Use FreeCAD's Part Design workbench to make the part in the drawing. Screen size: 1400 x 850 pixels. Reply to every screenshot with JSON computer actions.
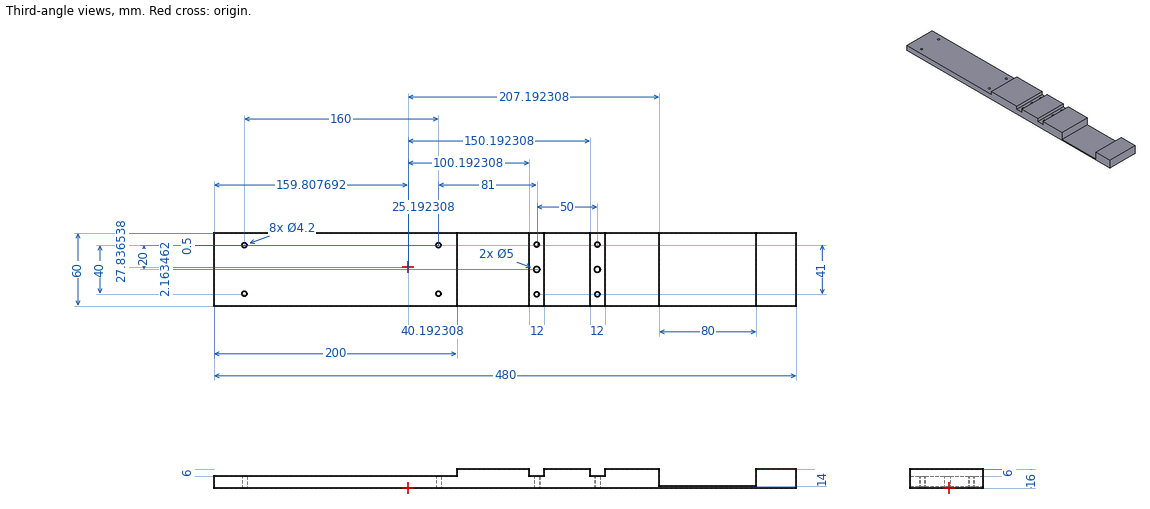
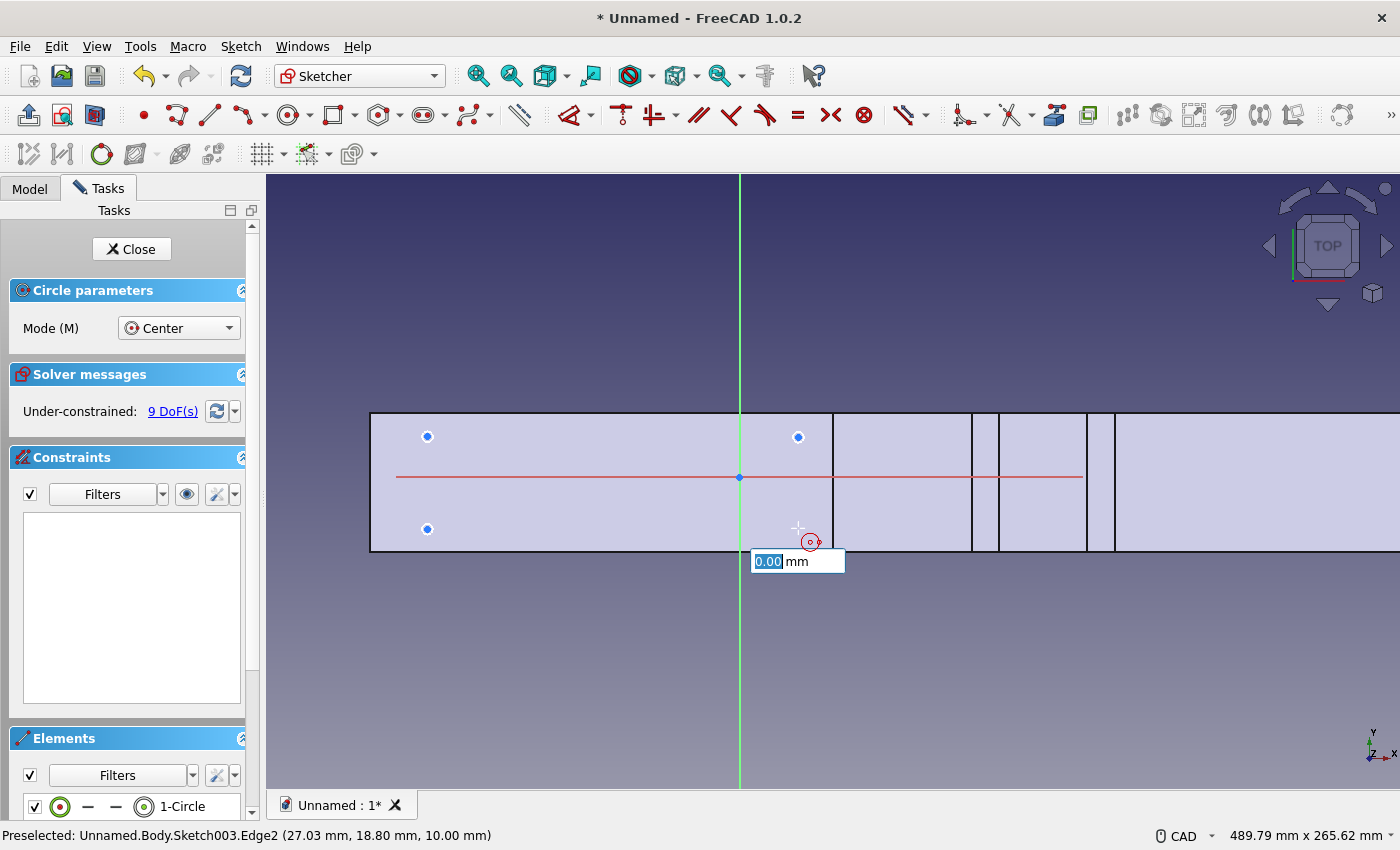
{"action": "scroll", "coordinate": [801, 525], "scroll_direction": "up", "scroll_amount": 6}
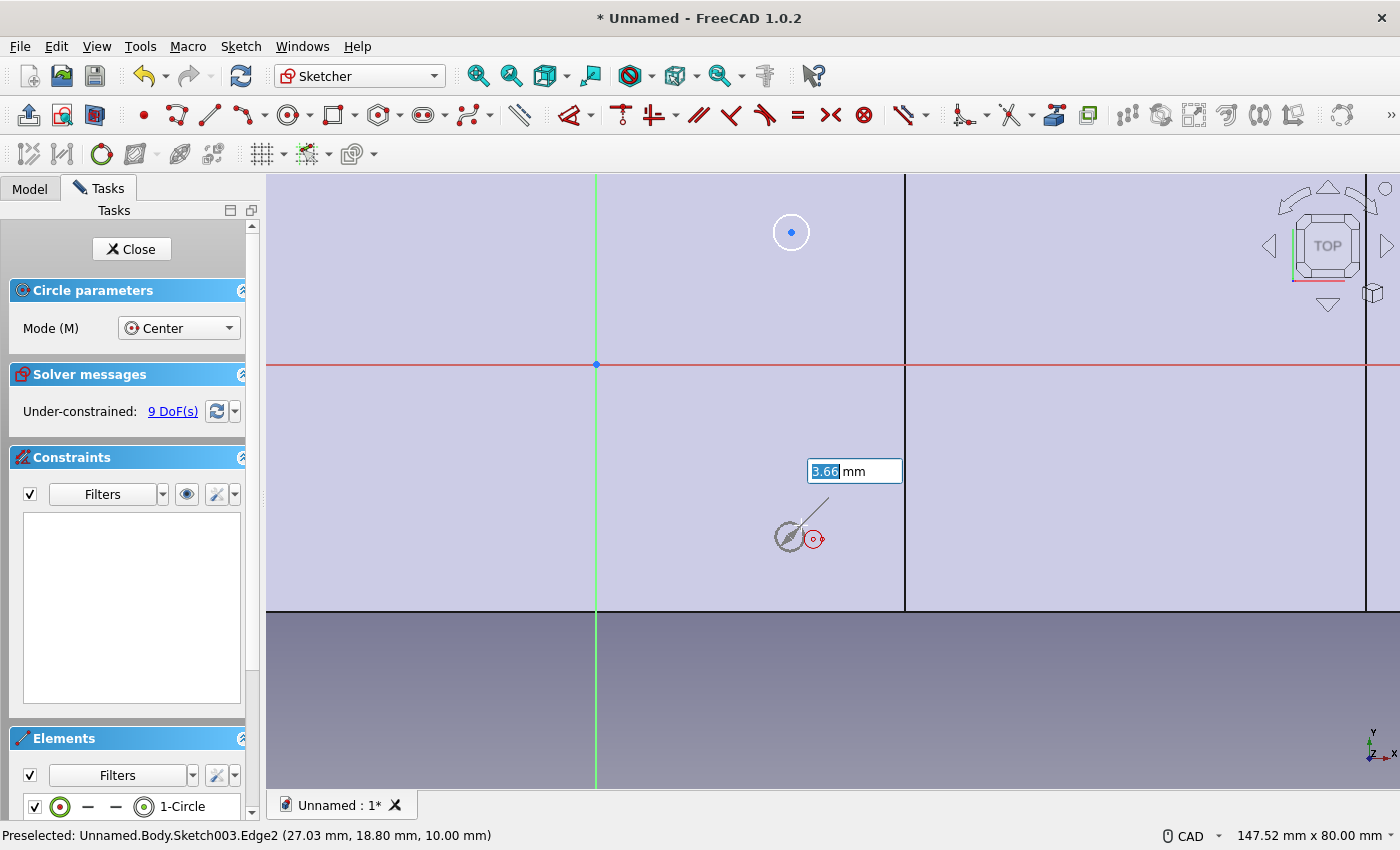
{"action": "left_click", "coordinate": [801, 524]}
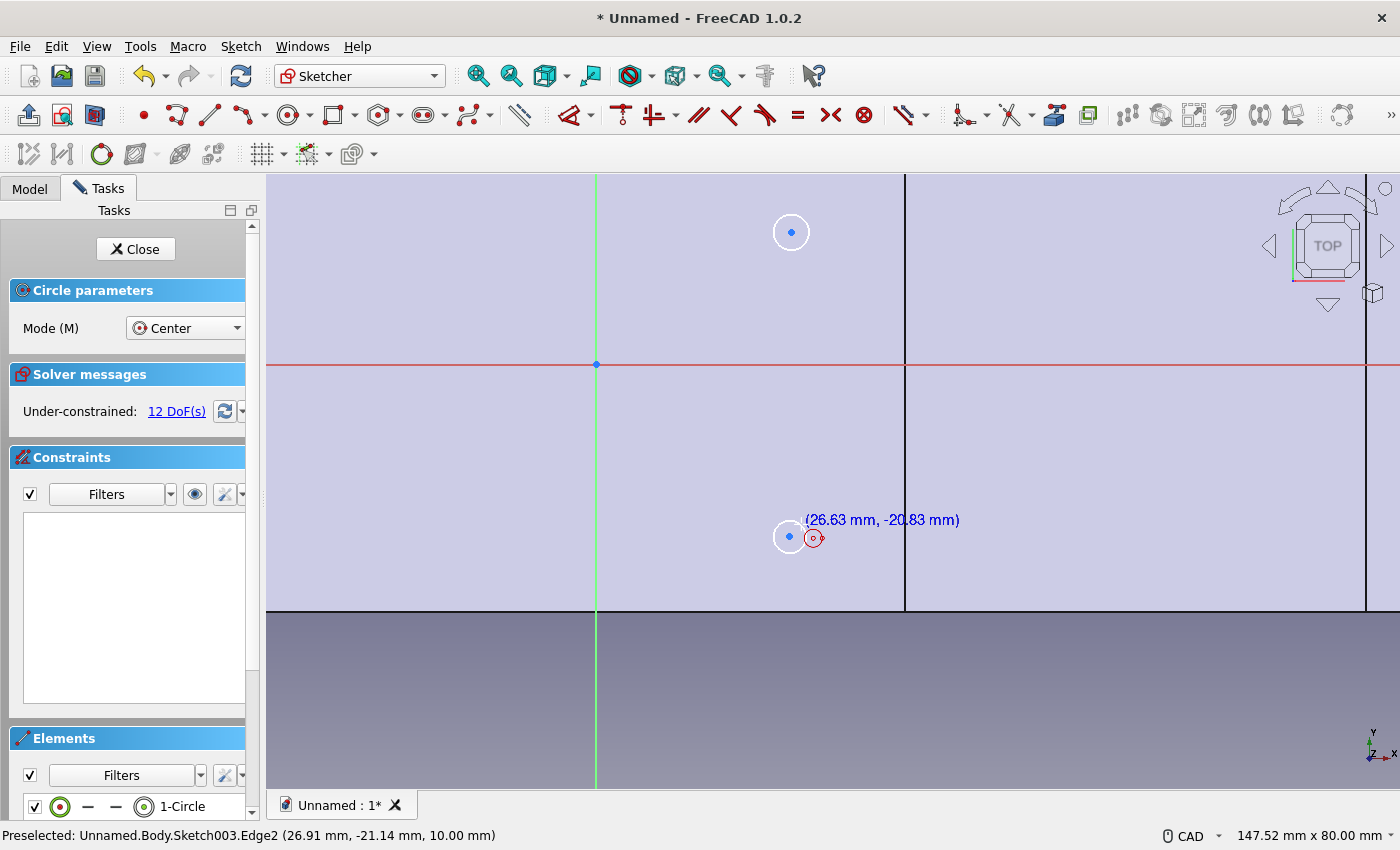
{"action": "scroll", "coordinate": [801, 525], "scroll_direction": "down", "scroll_amount": 6}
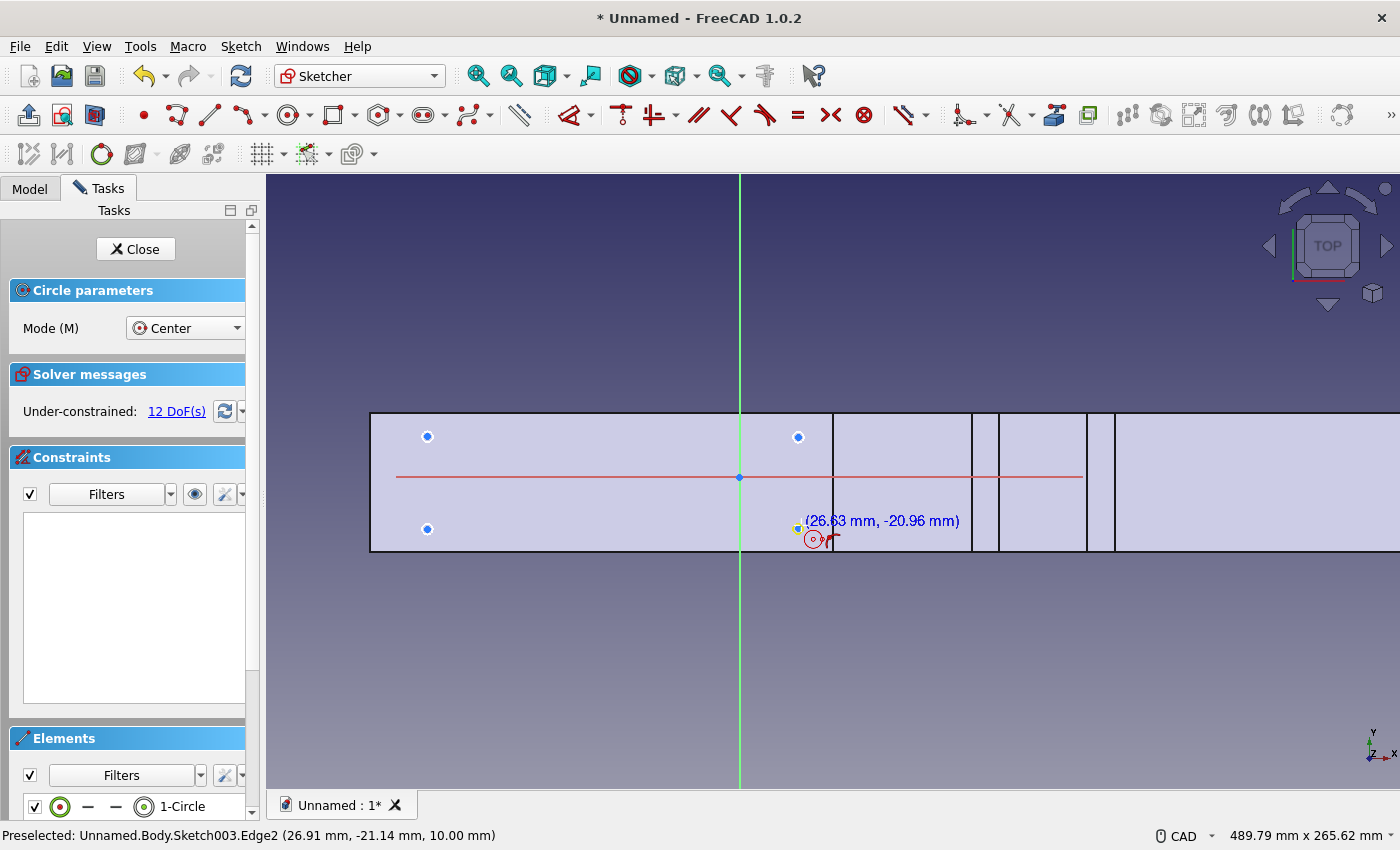
{"action": "scroll", "coordinate": [986, 435], "scroll_direction": "up", "scroll_amount": 8}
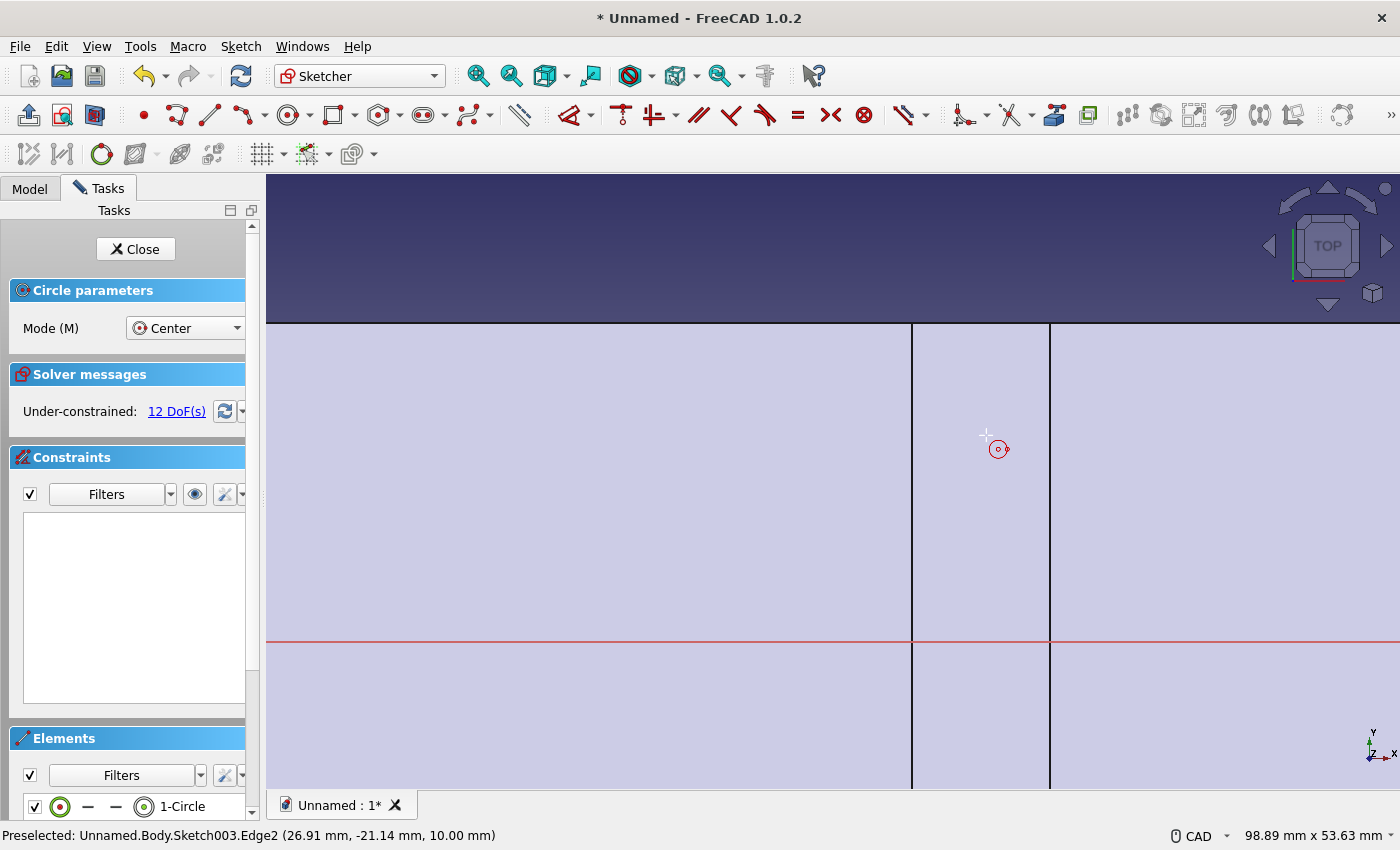
{"action": "scroll", "coordinate": [986, 435], "scroll_direction": "down", "scroll_amount": 8}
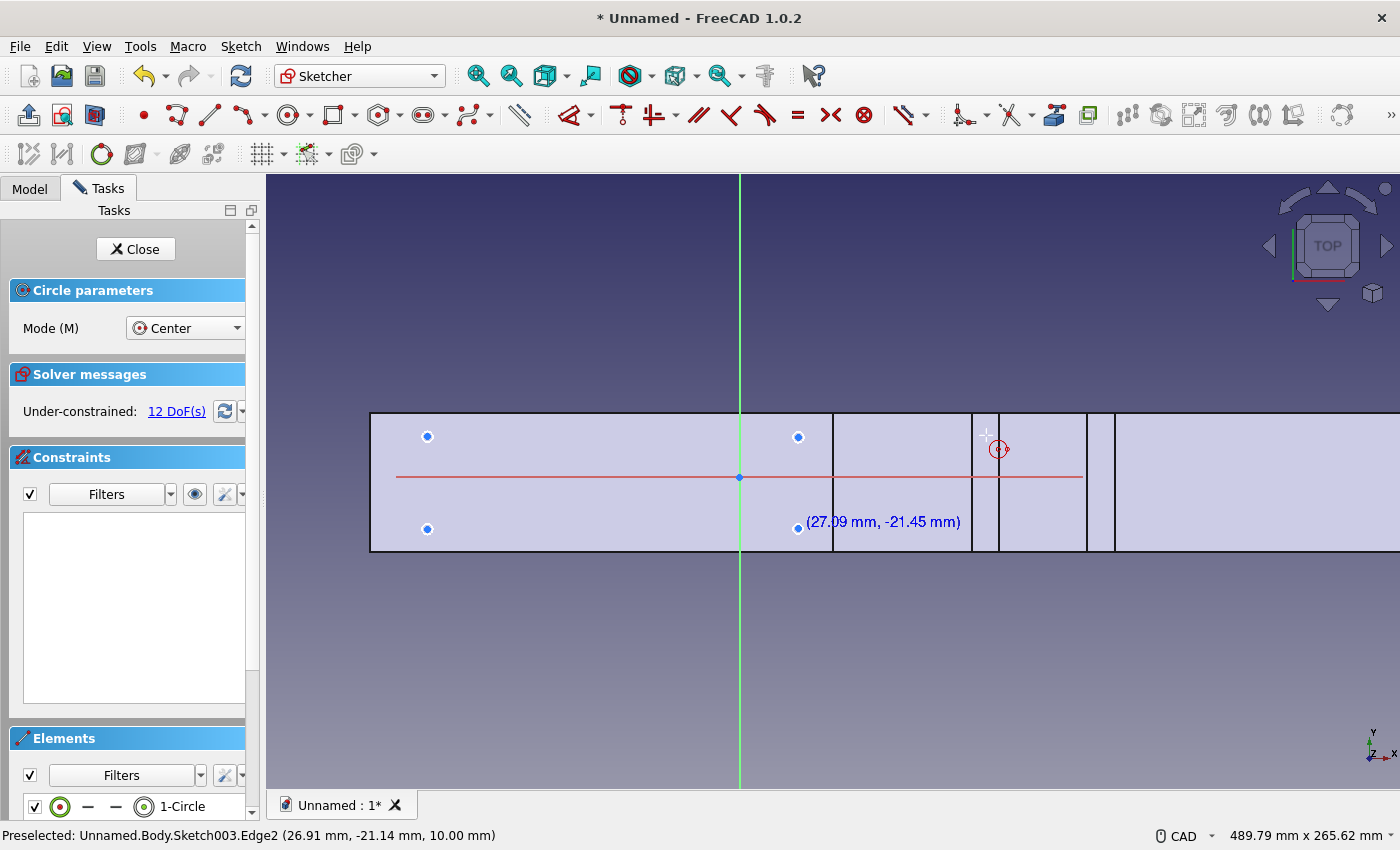
{"action": "left_click", "coordinate": [986, 435]}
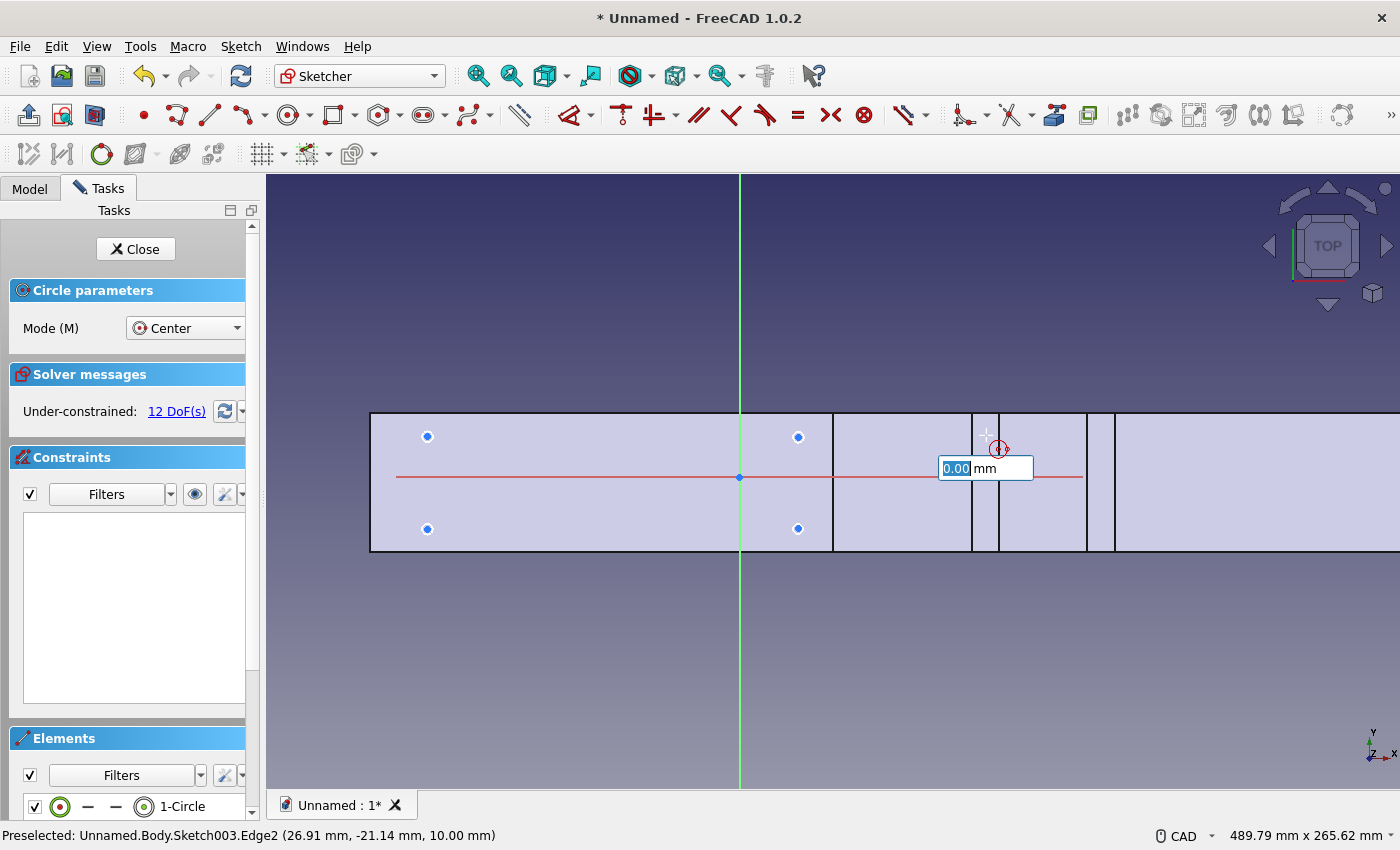
{"action": "scroll", "coordinate": [989, 431], "scroll_direction": "up", "scroll_amount": 6}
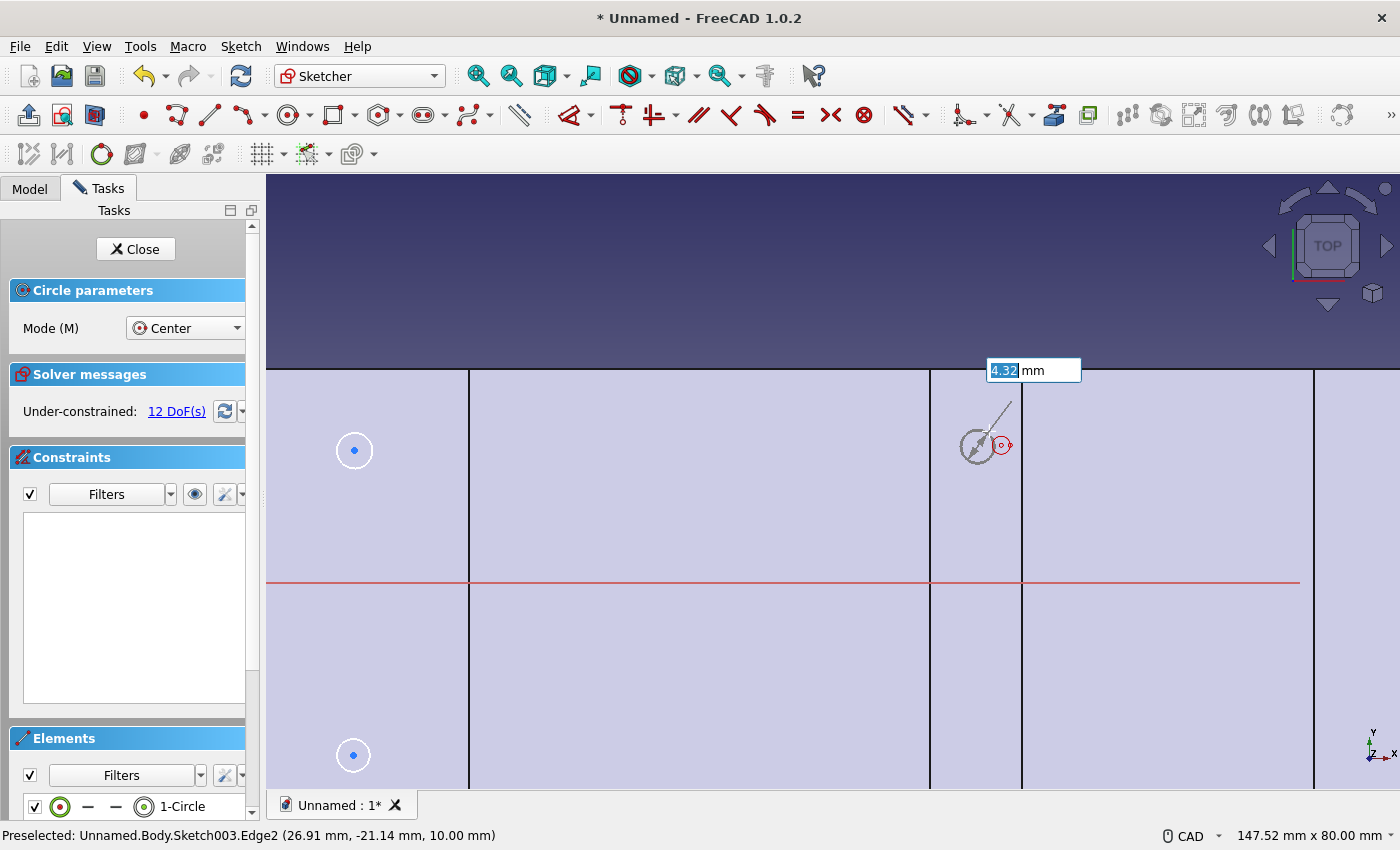
{"action": "left_click", "coordinate": [987, 431]}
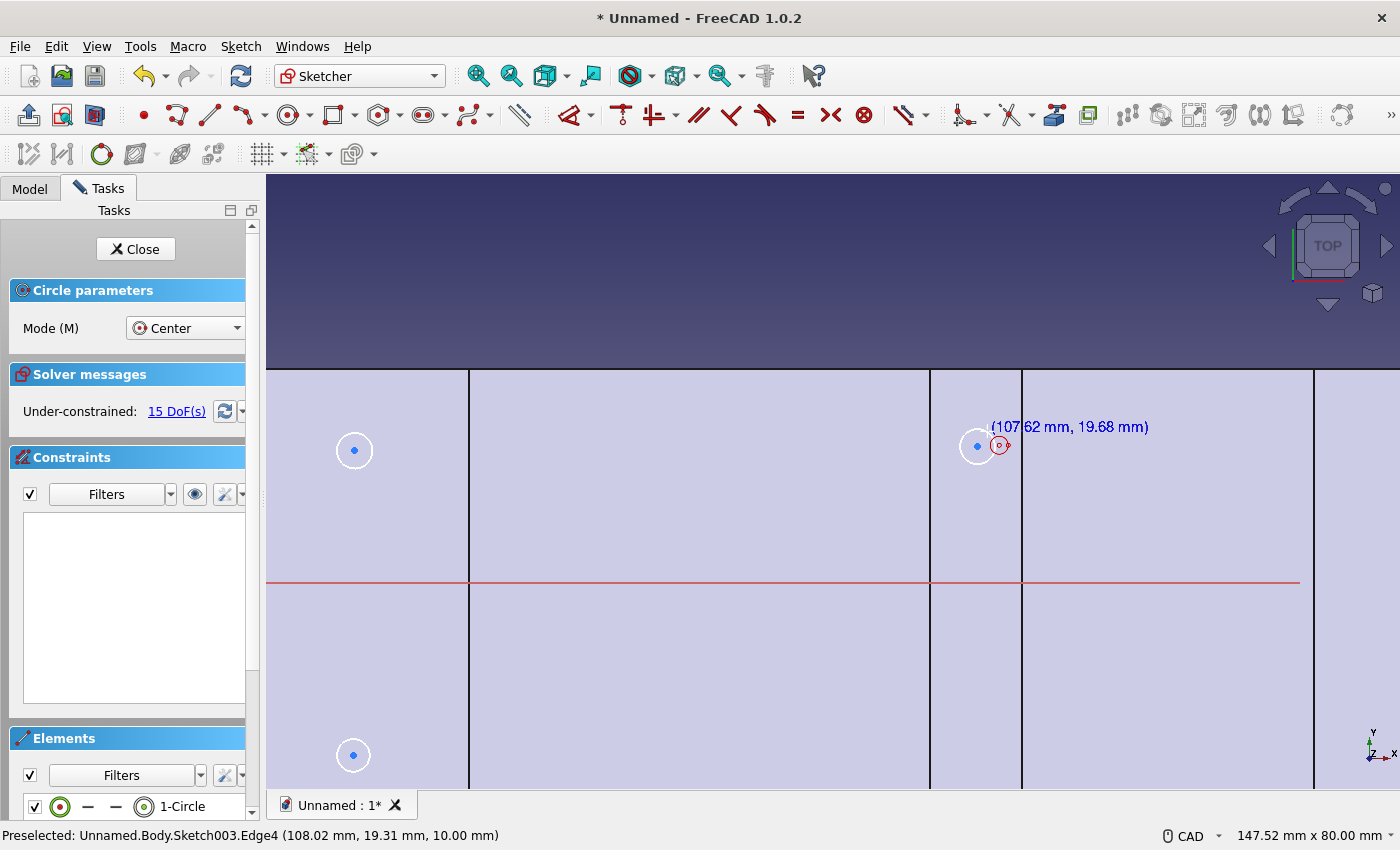
{"action": "scroll", "coordinate": [976, 758], "scroll_direction": "up", "scroll_amount": 2}